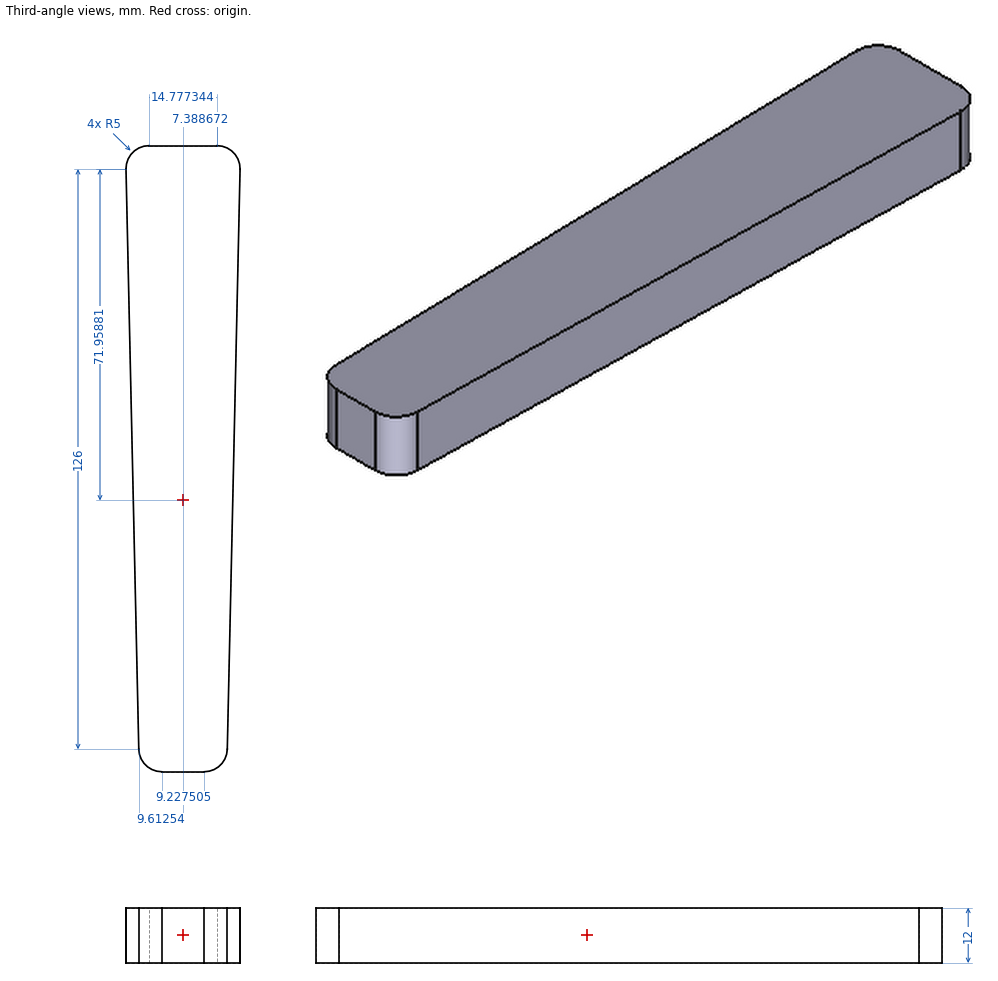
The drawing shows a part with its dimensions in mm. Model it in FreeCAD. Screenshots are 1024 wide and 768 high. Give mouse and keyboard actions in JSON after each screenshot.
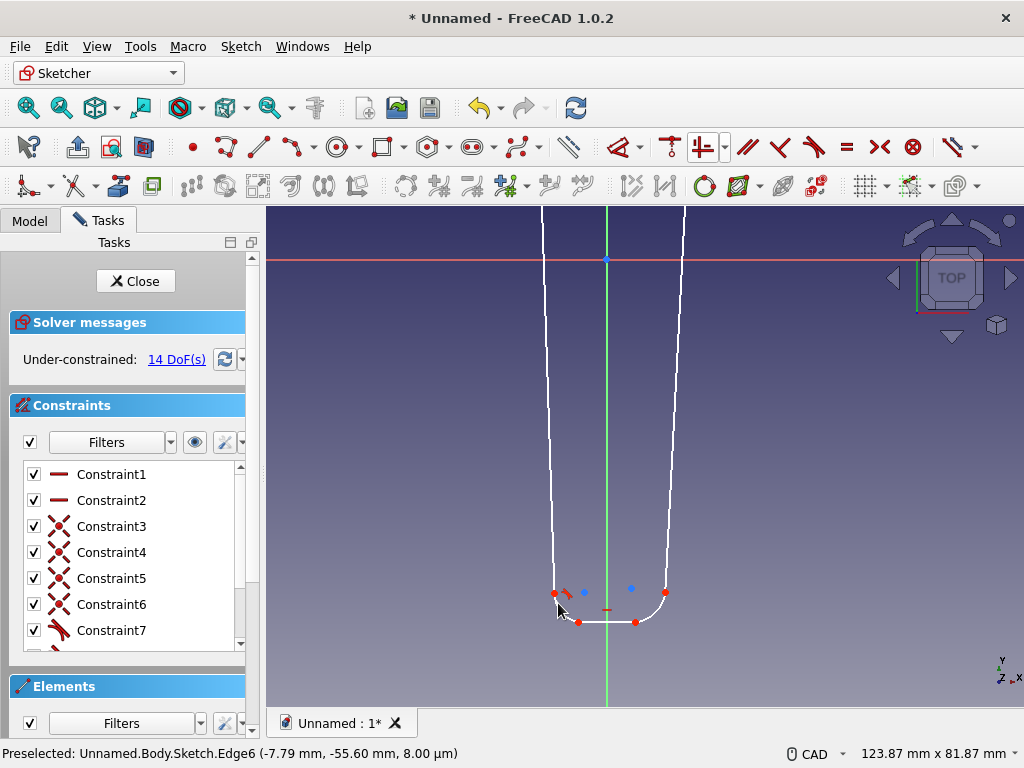
{"action": "scroll", "coordinate": [596, 622], "scroll_direction": "up", "scroll_amount": 2}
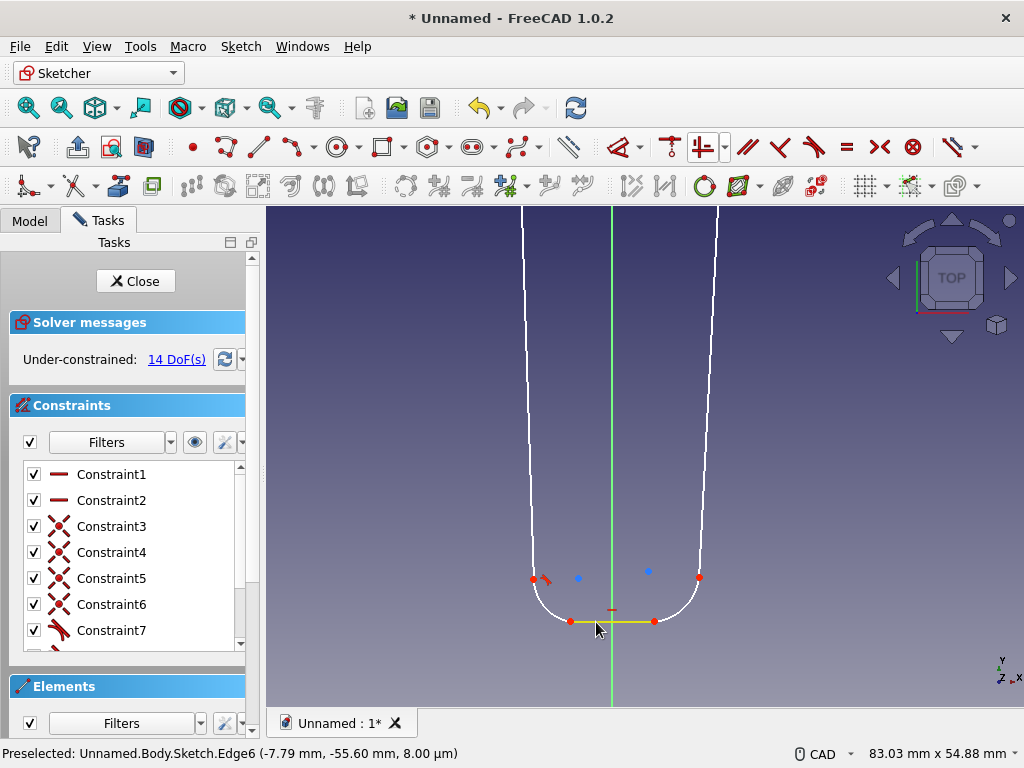
{"action": "left_click", "coordinate": [596, 622]}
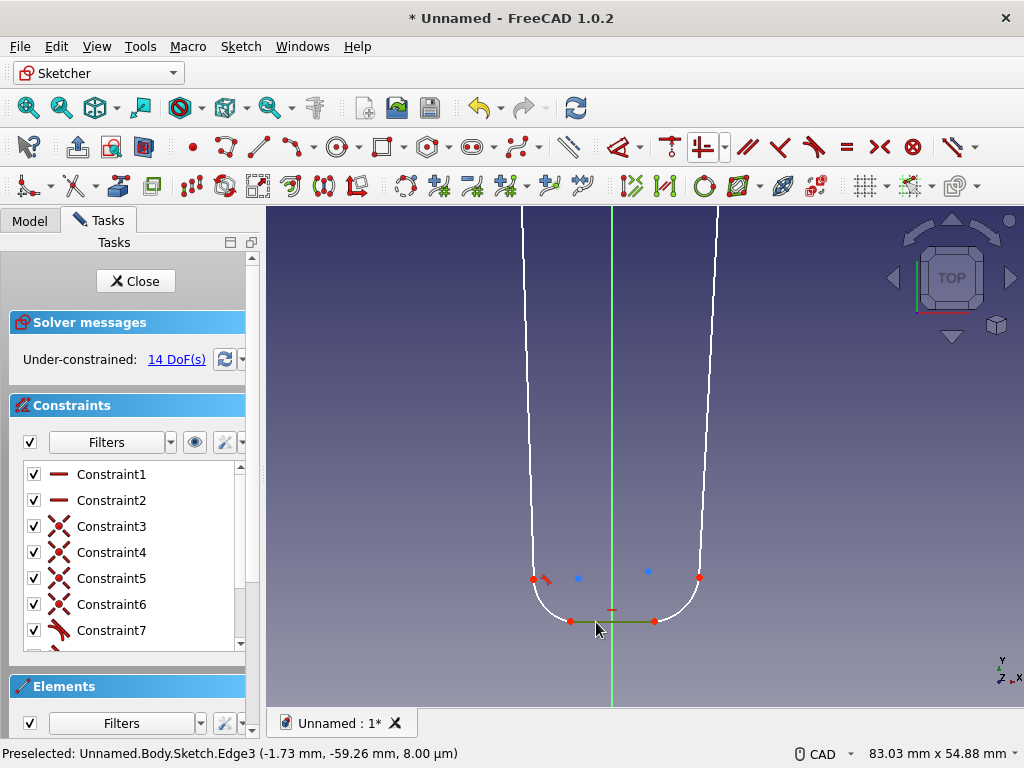
{"action": "left_click", "coordinate": [538, 597]}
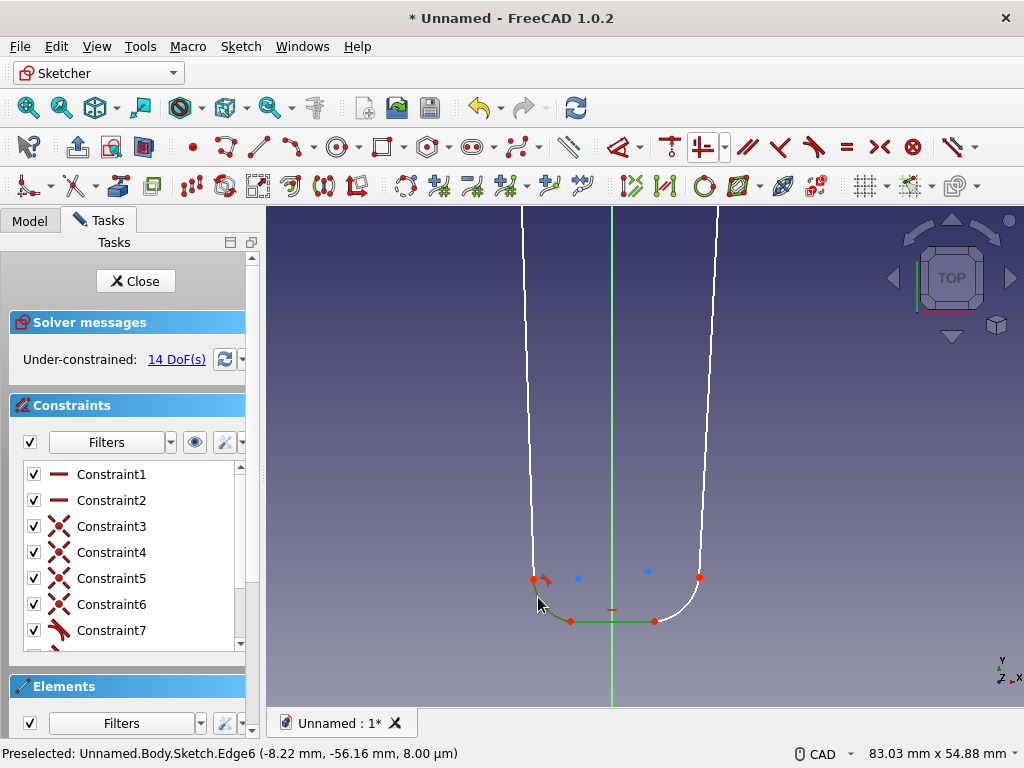
{"action": "left_click", "coordinate": [814, 148]}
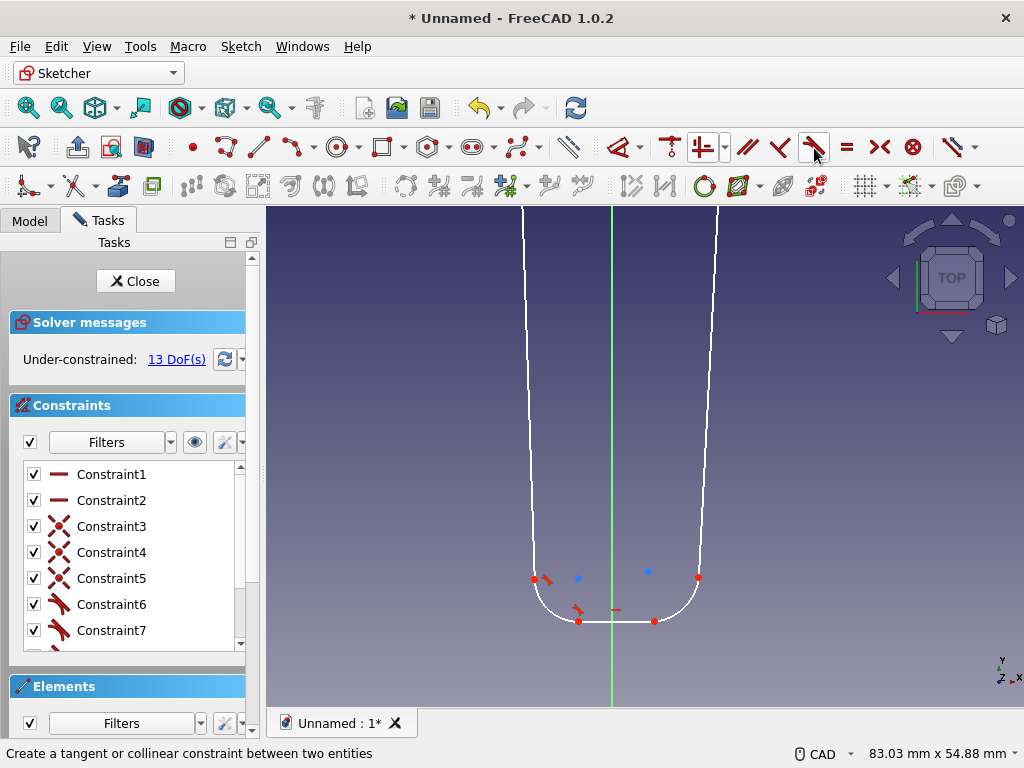
{"action": "scroll", "coordinate": [601, 622], "scroll_direction": "up", "scroll_amount": 2}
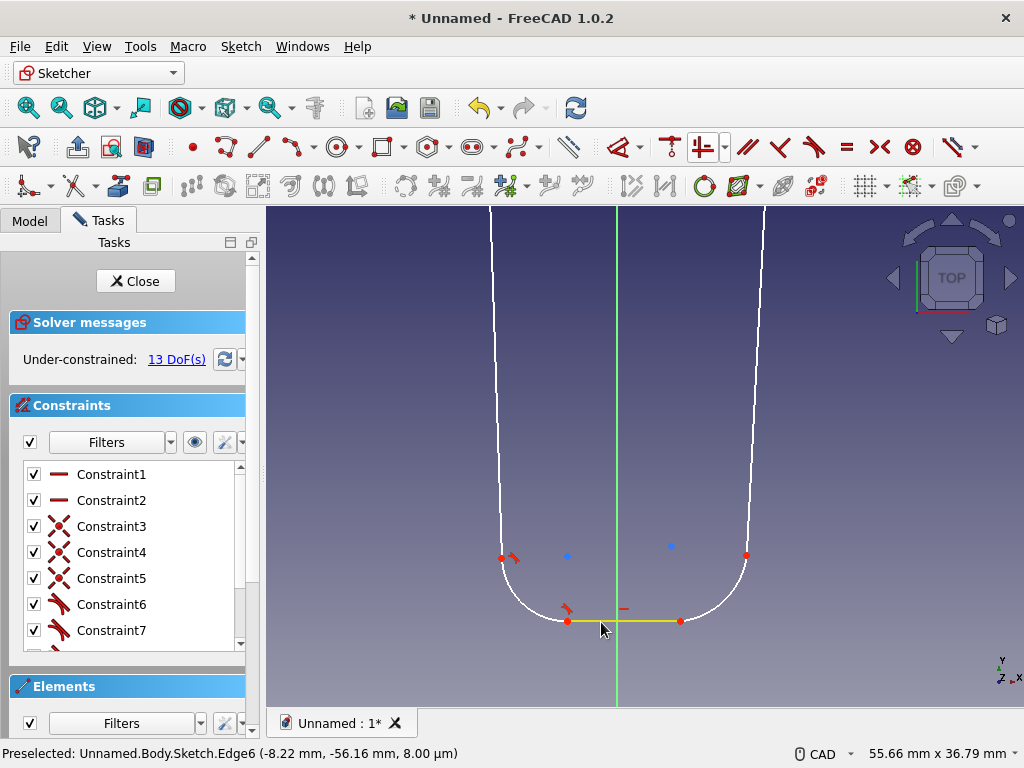
{"action": "left_click", "coordinate": [601, 621]}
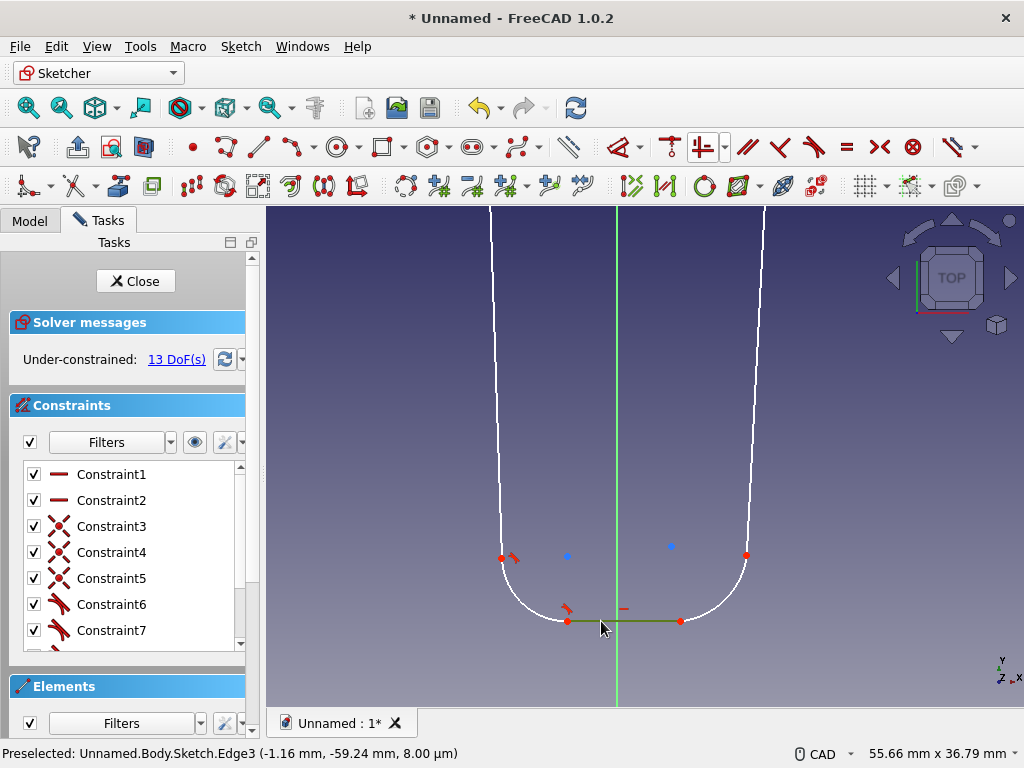
{"action": "left_click", "coordinate": [709, 612]}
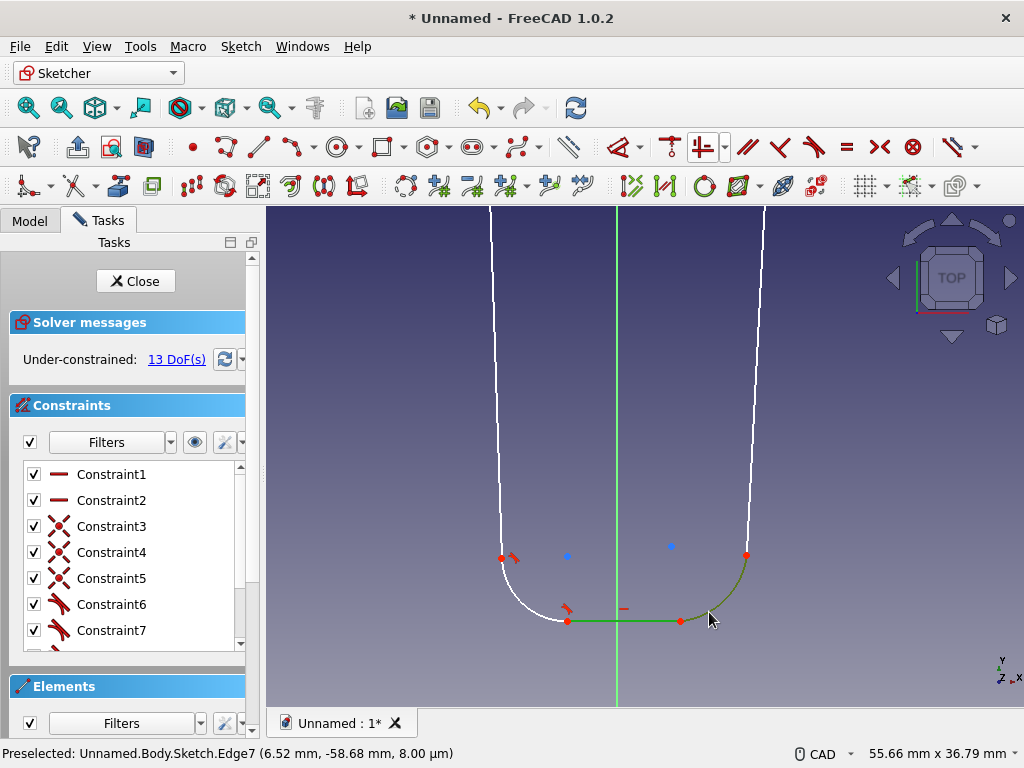
{"action": "key", "text": "t"}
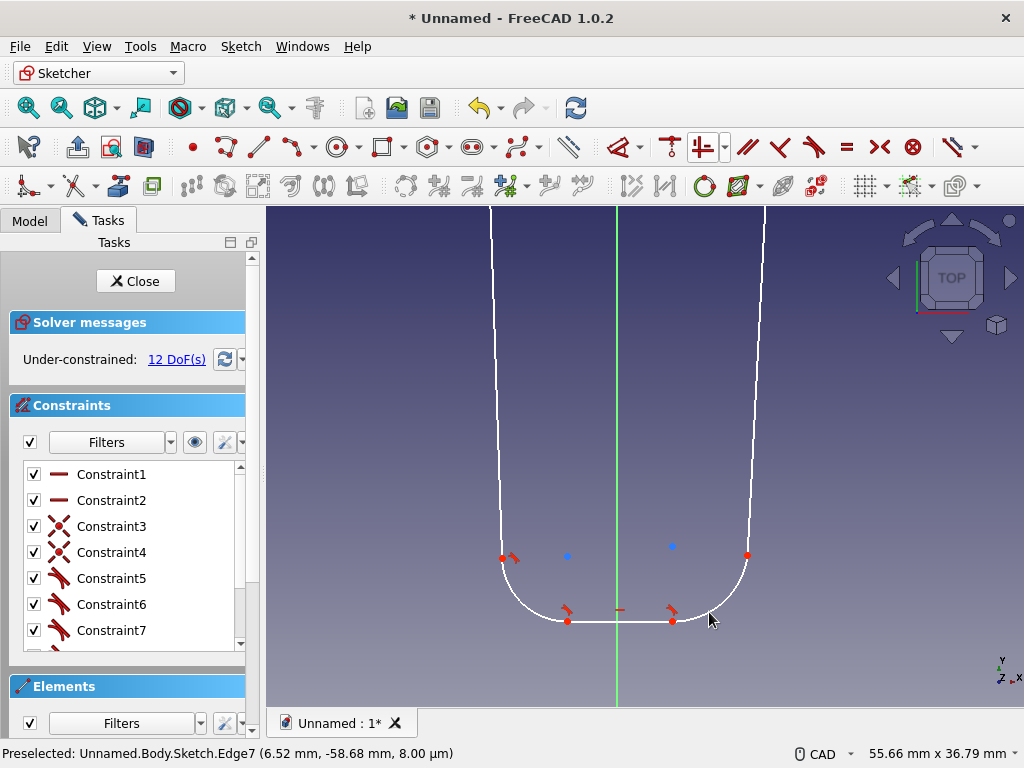
{"action": "scroll", "coordinate": [569, 608], "scroll_direction": "down", "scroll_amount": 9}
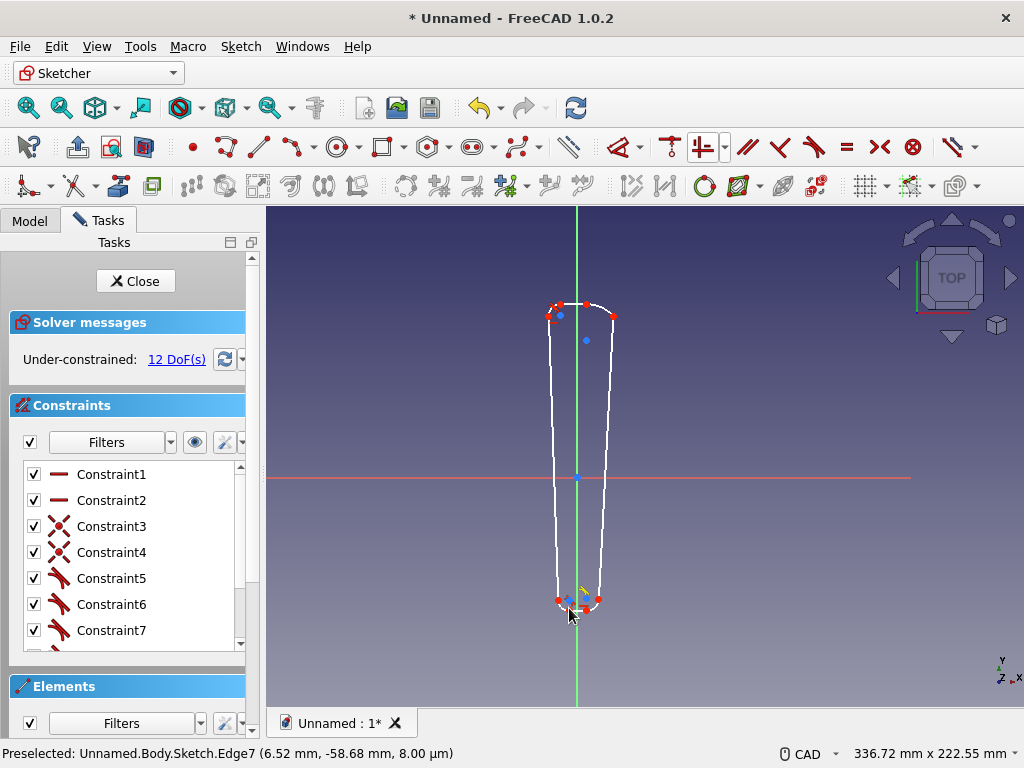
{"action": "left_click", "coordinate": [603, 515]}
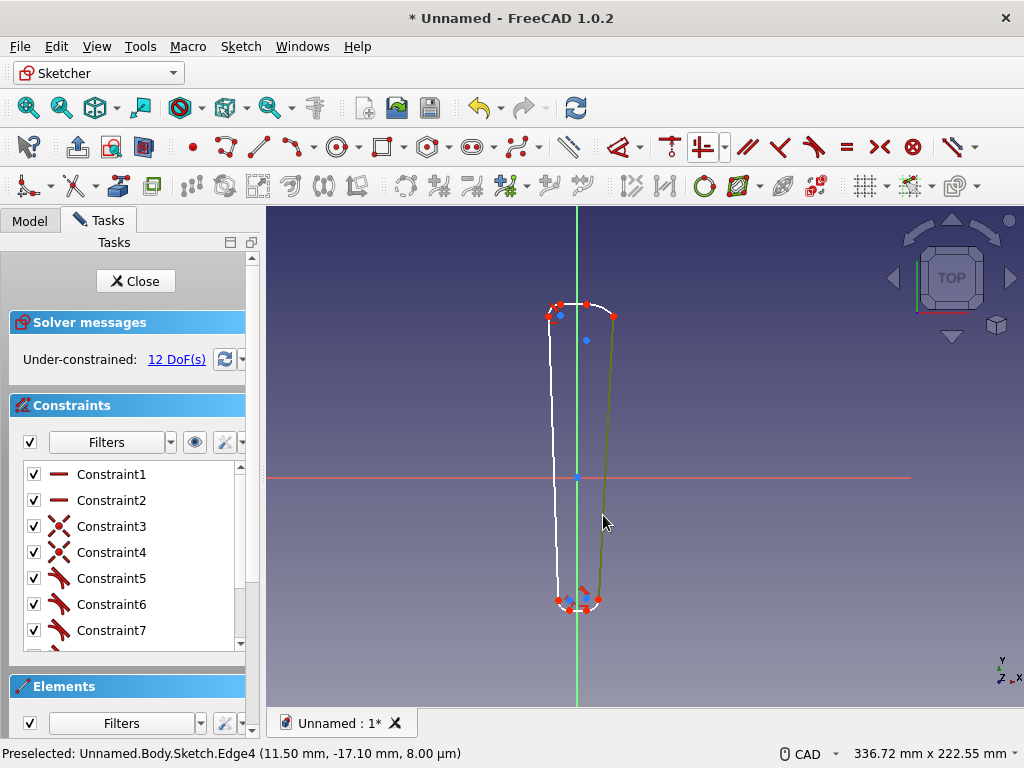
{"action": "scroll", "coordinate": [595, 608], "scroll_direction": "up", "scroll_amount": 3}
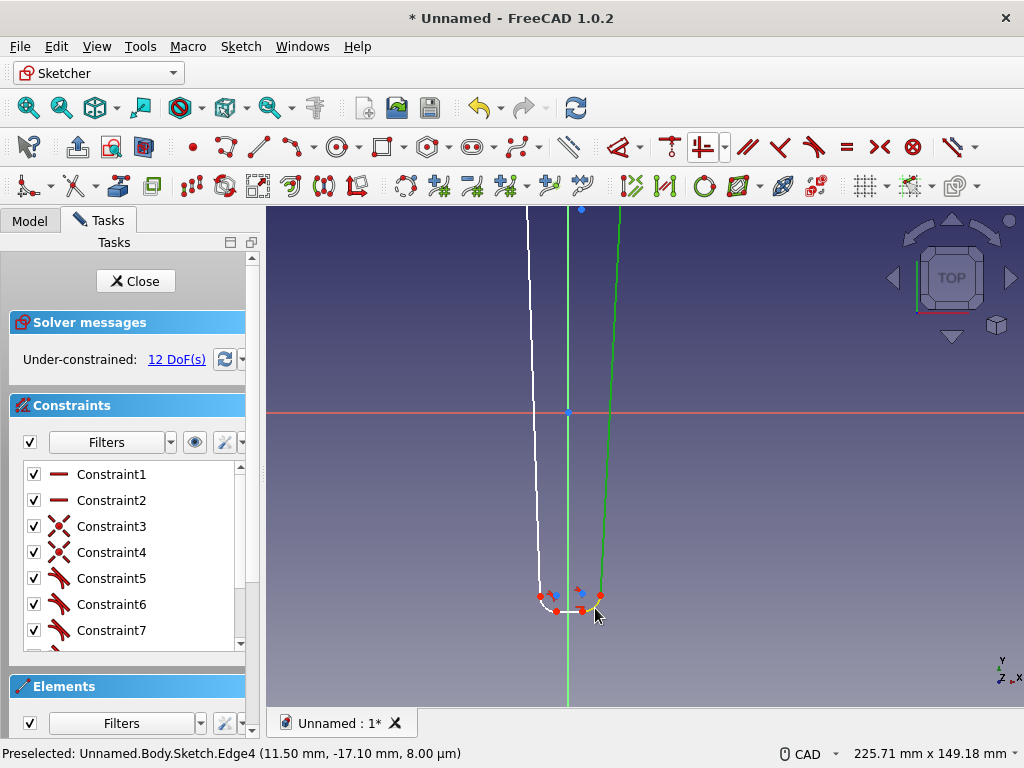
{"action": "left_click", "coordinate": [594, 607]}